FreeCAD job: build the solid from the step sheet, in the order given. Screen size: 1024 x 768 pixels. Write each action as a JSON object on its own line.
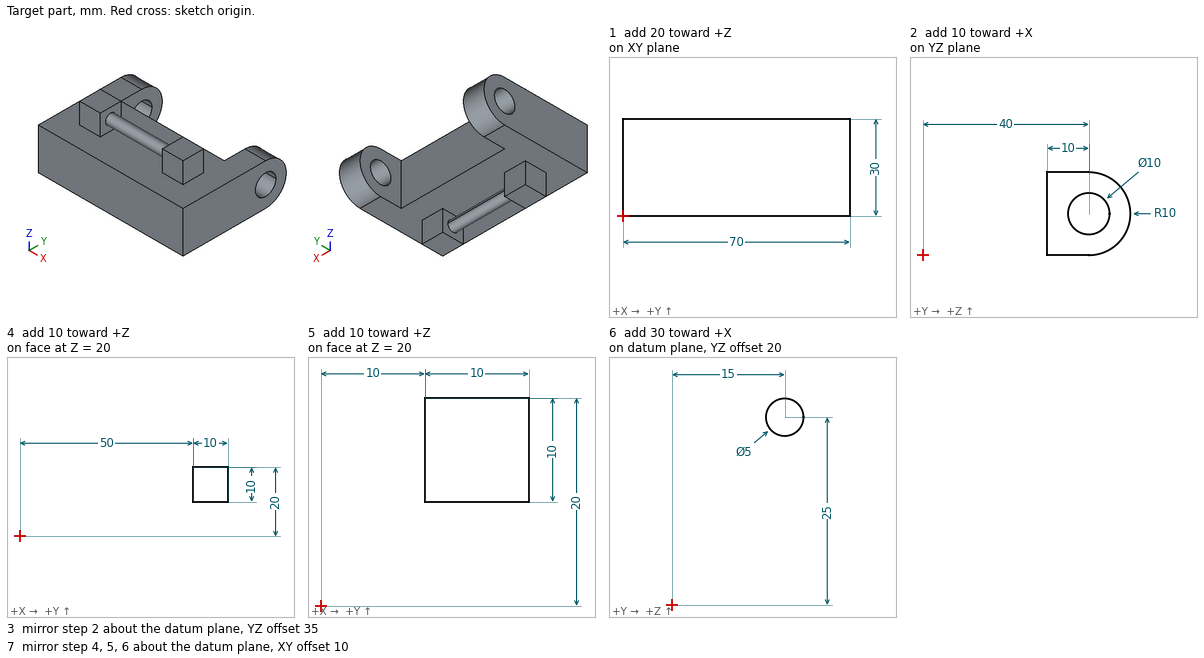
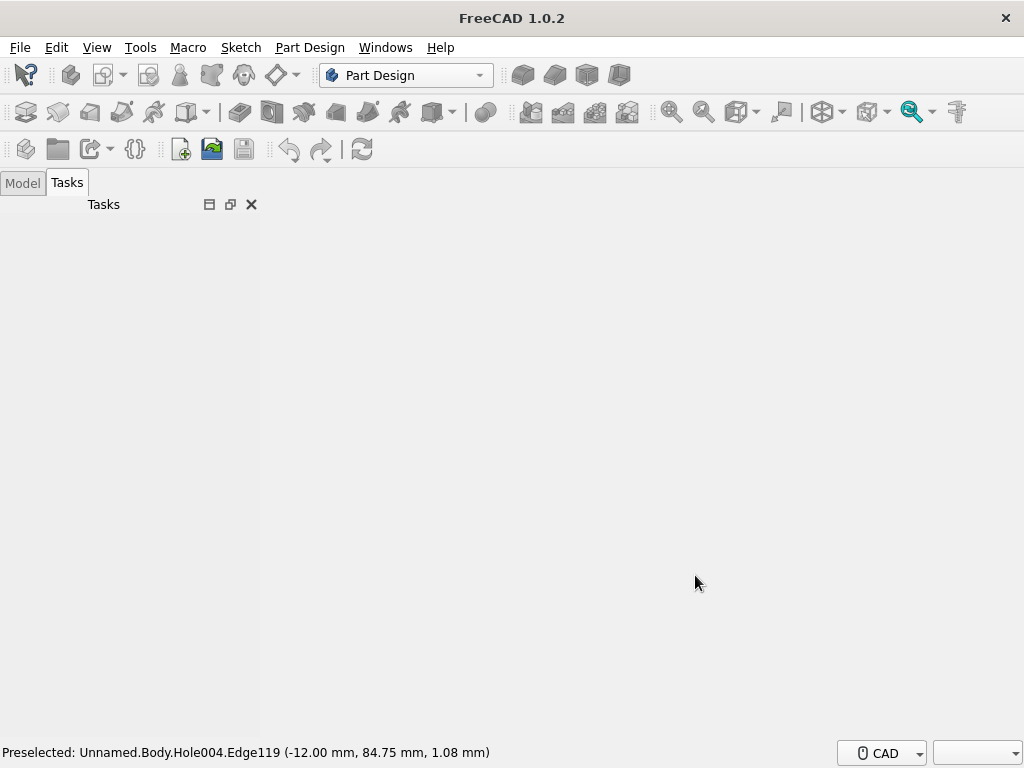
{"action": "key", "text": "ctrl+n"}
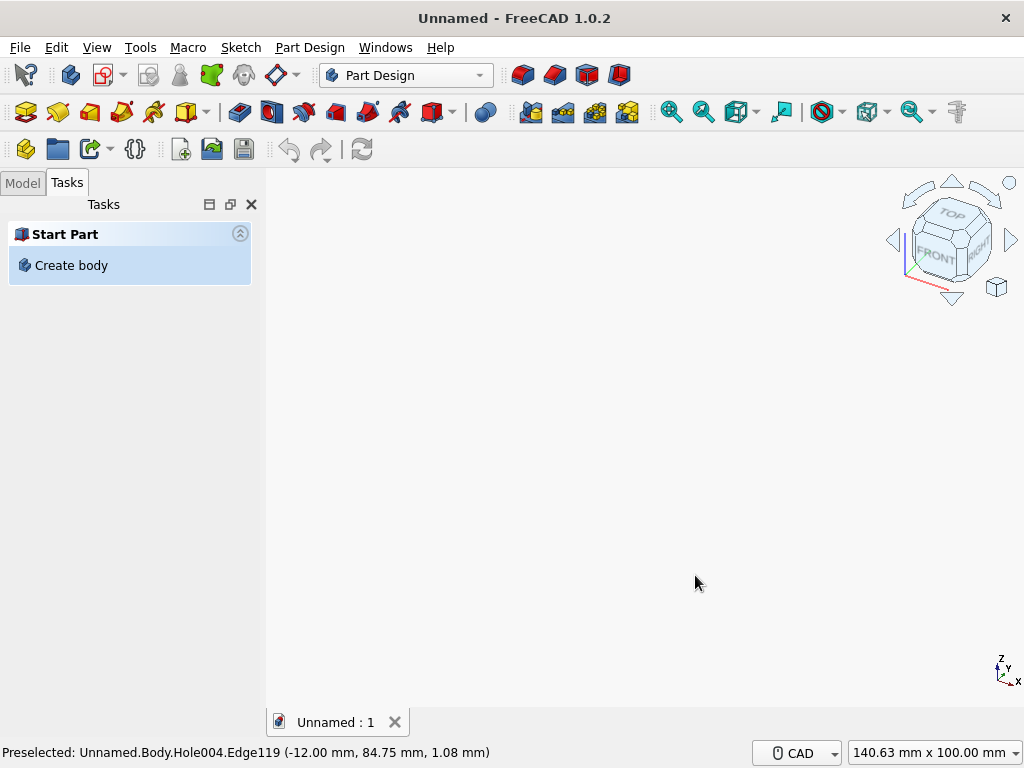
{"action": "left_click", "coordinate": [104, 76]}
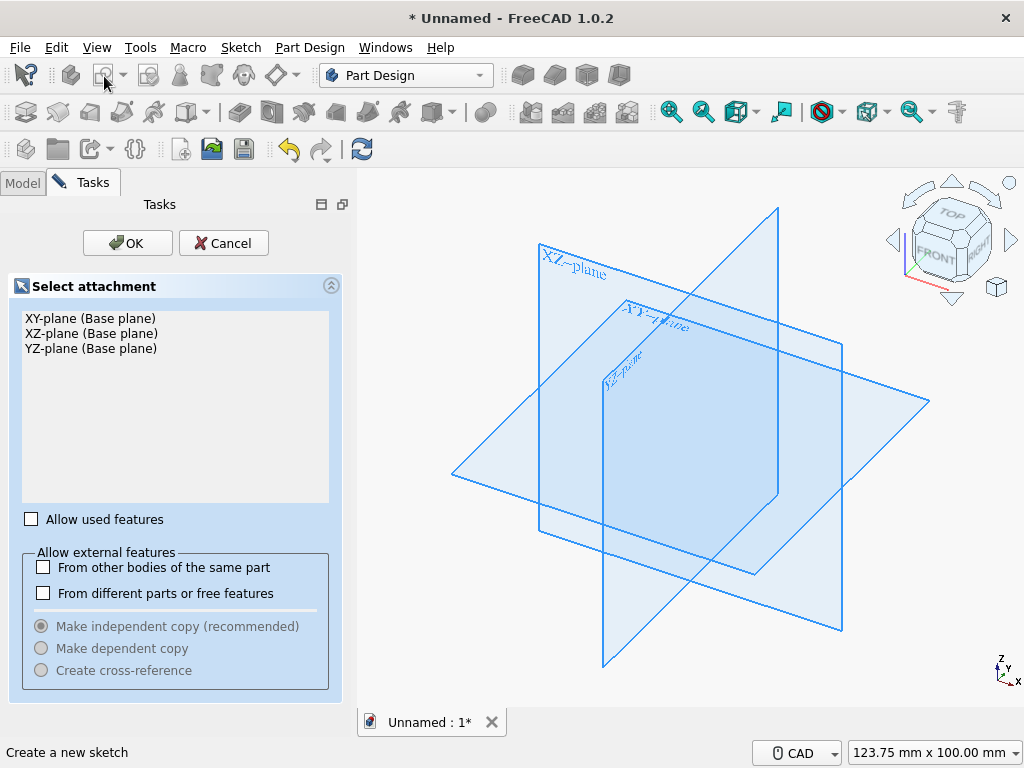
{"action": "left_click", "coordinate": [82, 318]}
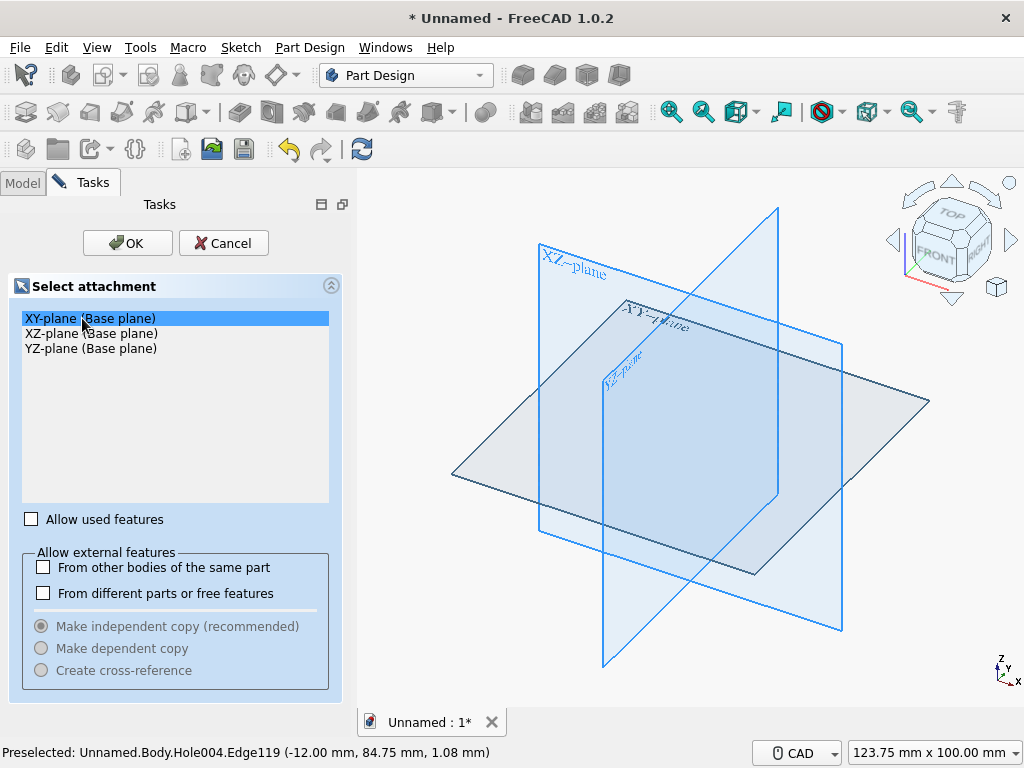
{"action": "left_click", "coordinate": [128, 243]}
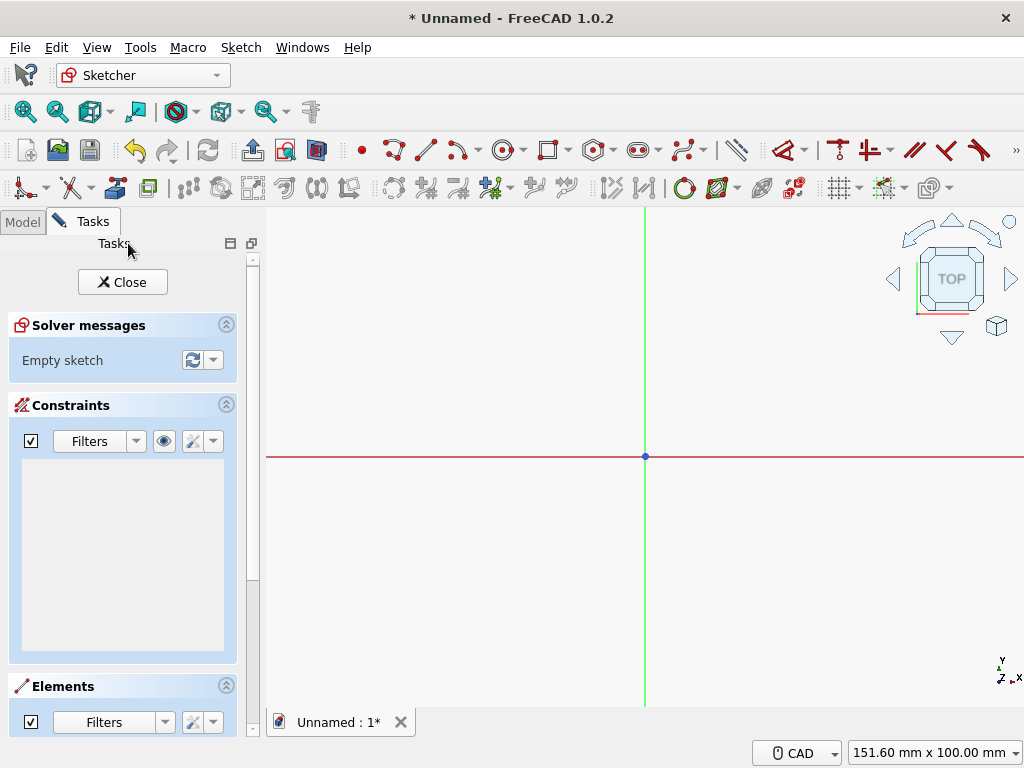
{"action": "scroll", "coordinate": [294, 609], "scroll_direction": "down", "scroll_amount": 2}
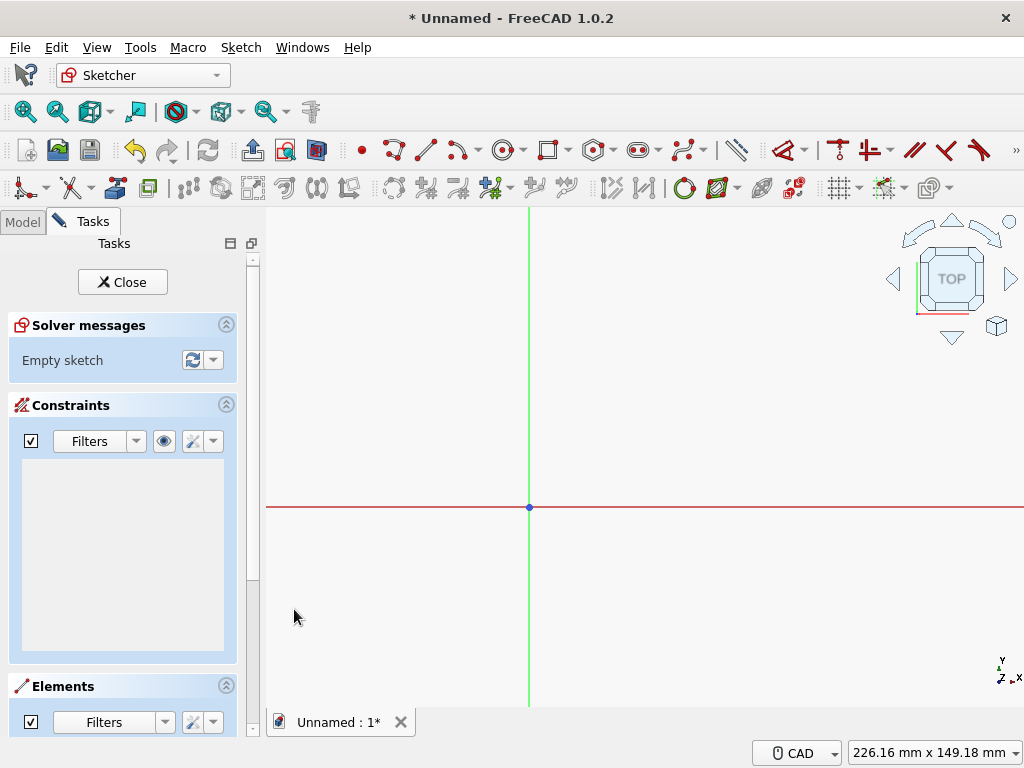
{"action": "scroll", "coordinate": [732, 457], "scroll_direction": "up", "scroll_amount": 3}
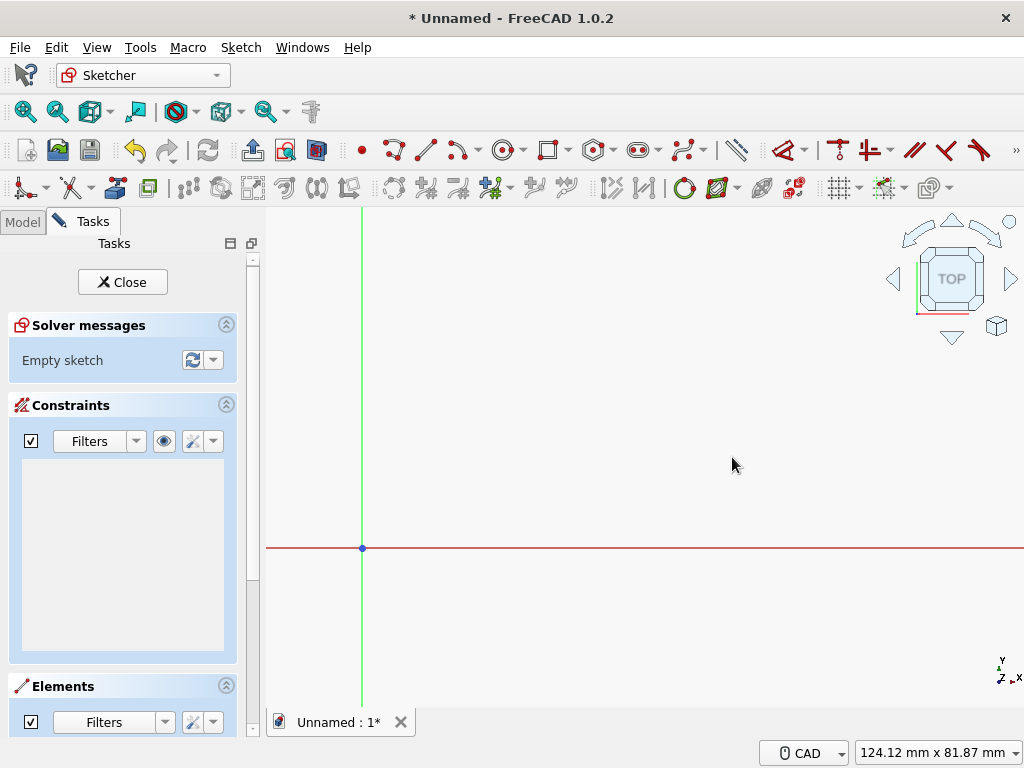
{"action": "key", "text": "g r"}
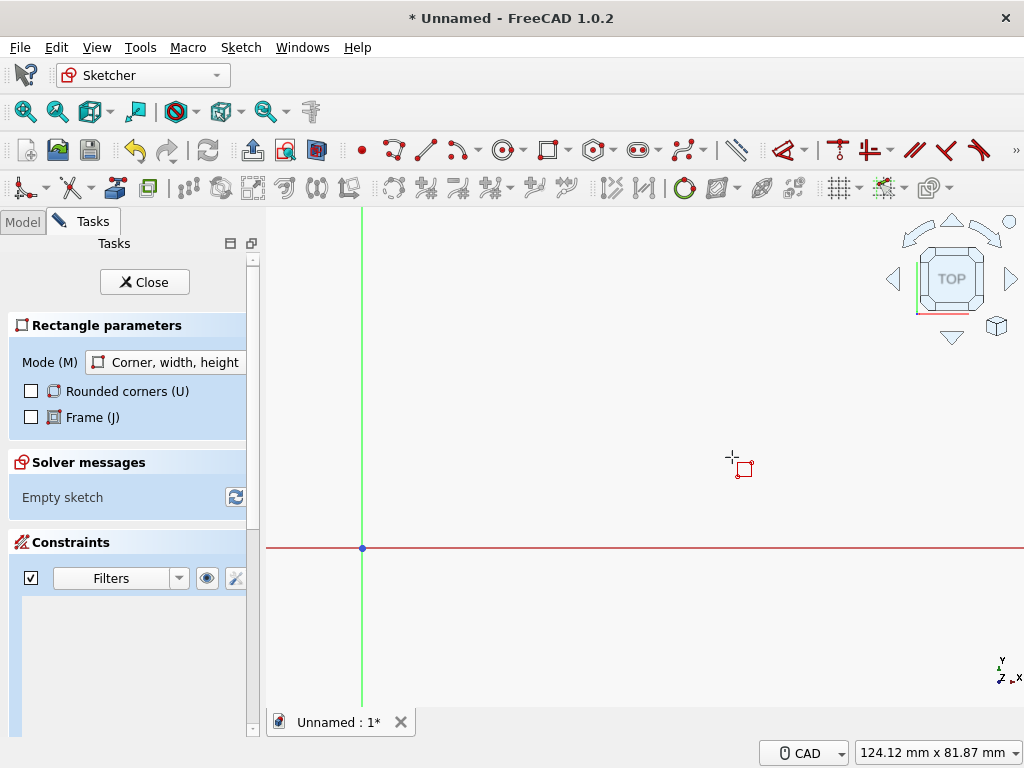
{"action": "left_click", "coordinate": [362, 548]}
{"action": "mouse_move", "coordinate": [790, 365]}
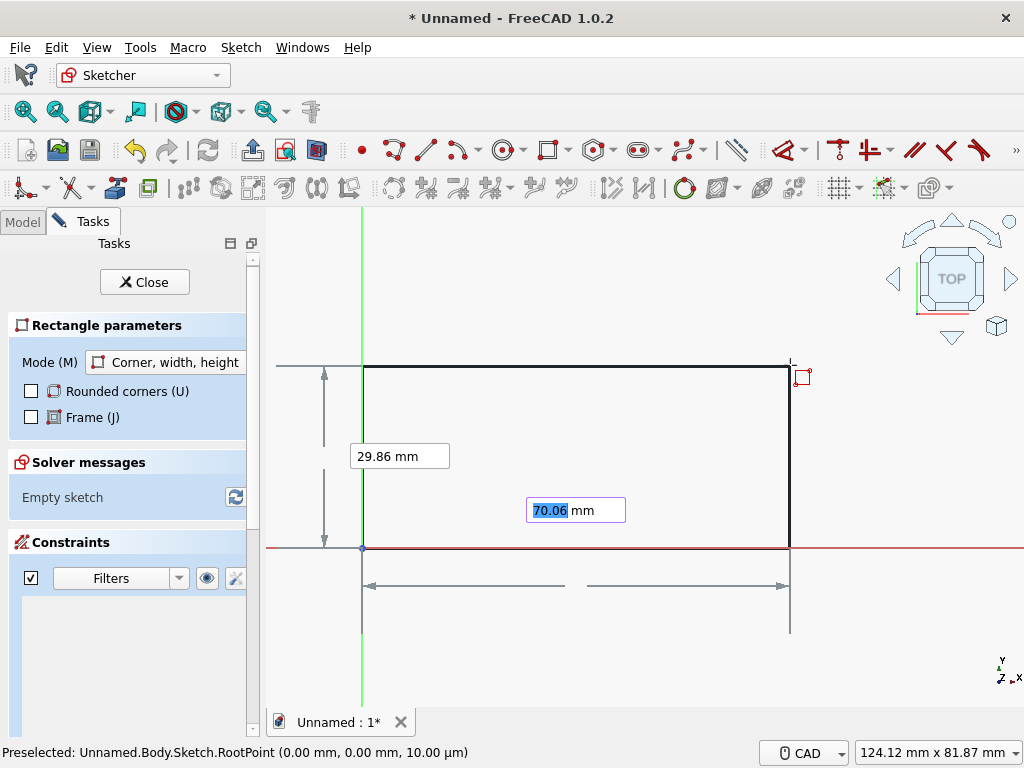
{"action": "type", "text": "70"}
{"action": "key", "text": "Tab"}
{"action": "type", "text": "30"}
{"action": "key", "text": "Return"}
{"action": "key", "text": "Escape"}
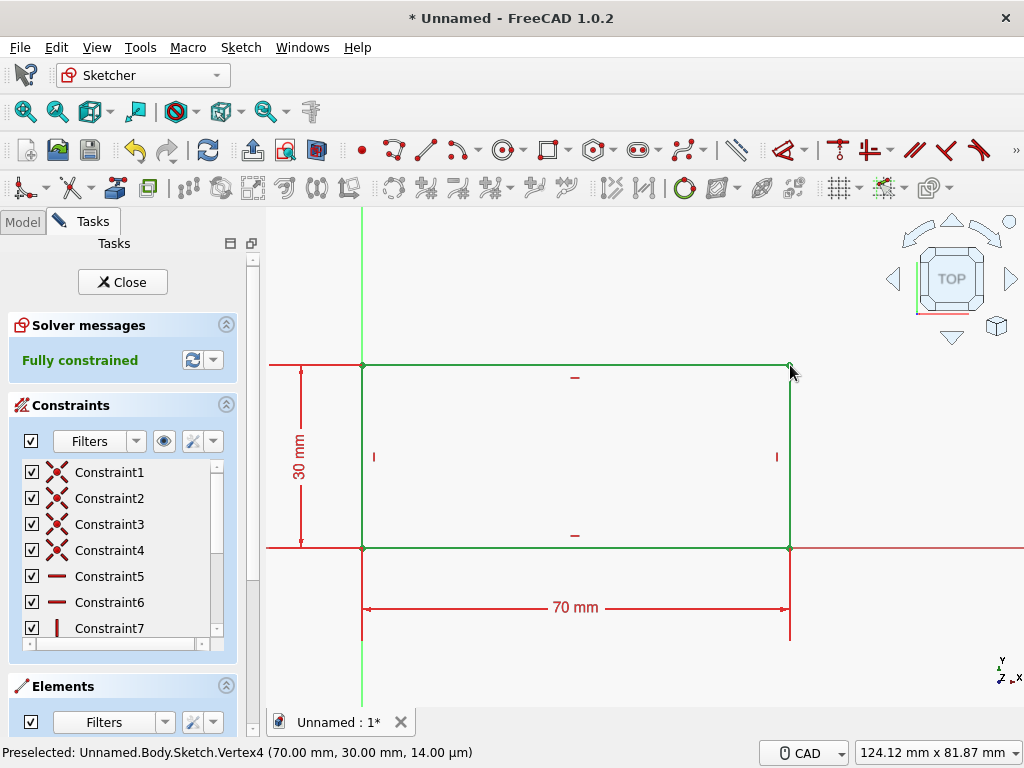
{"action": "left_click", "coordinate": [123, 282]}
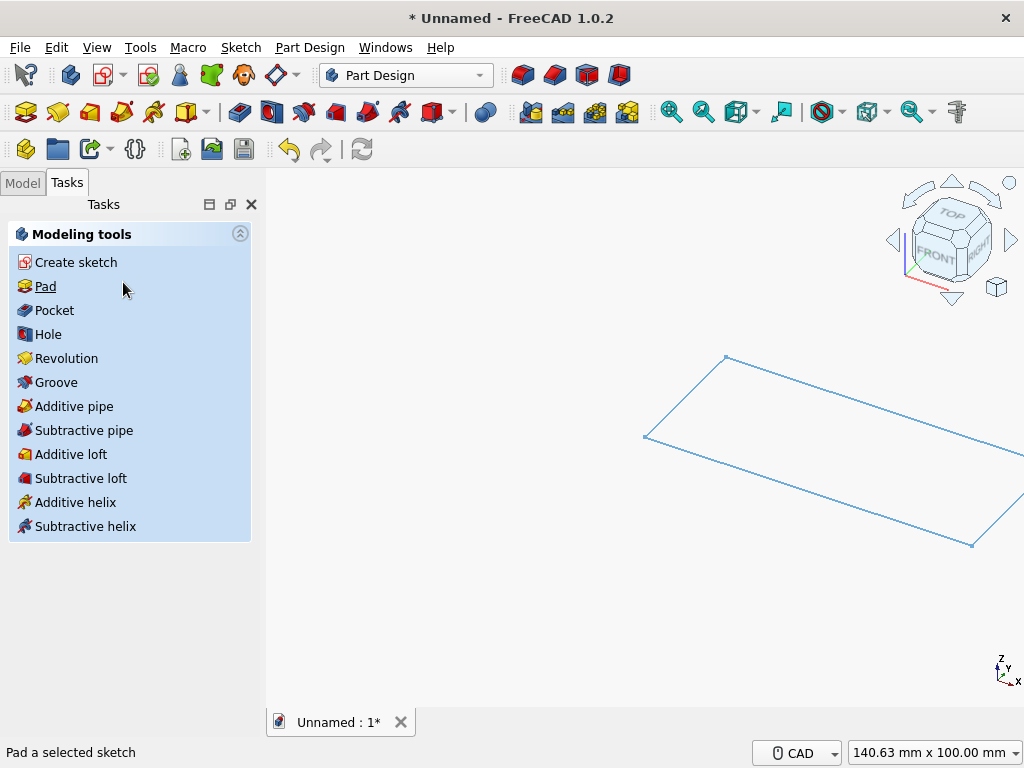
{"action": "left_click", "coordinate": [26, 112]}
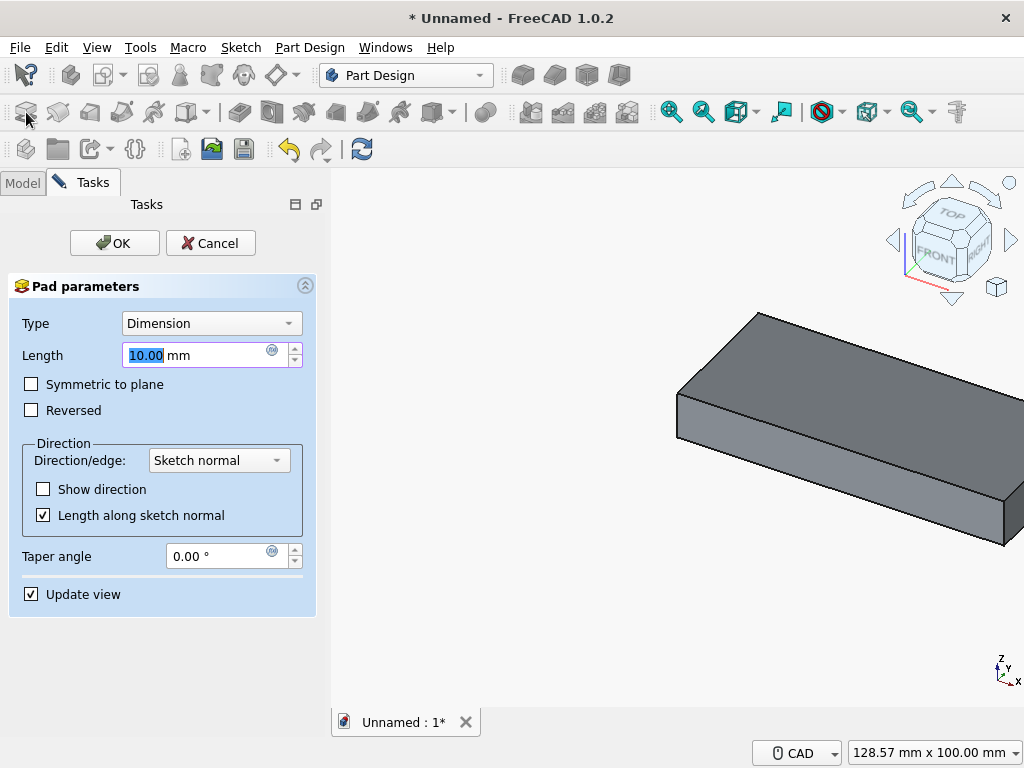
{"action": "type", "text": "20"}
{"action": "key", "text": "Tab"}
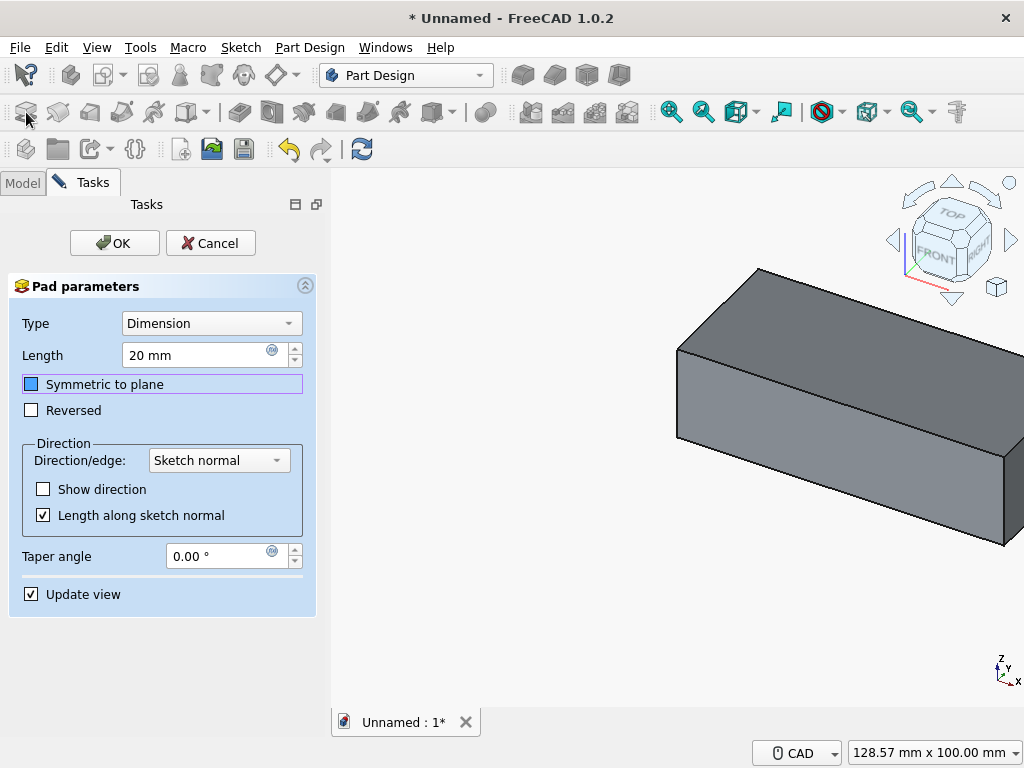
{"action": "left_click", "coordinate": [115, 243]}